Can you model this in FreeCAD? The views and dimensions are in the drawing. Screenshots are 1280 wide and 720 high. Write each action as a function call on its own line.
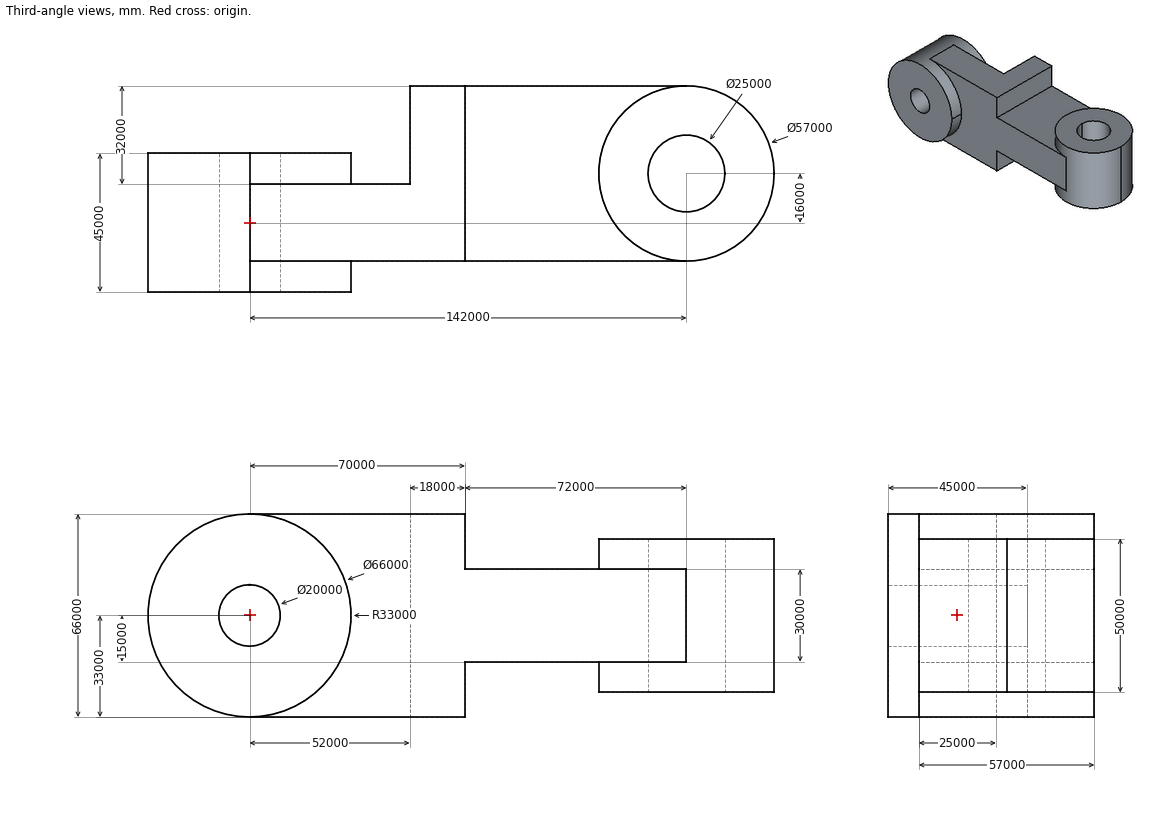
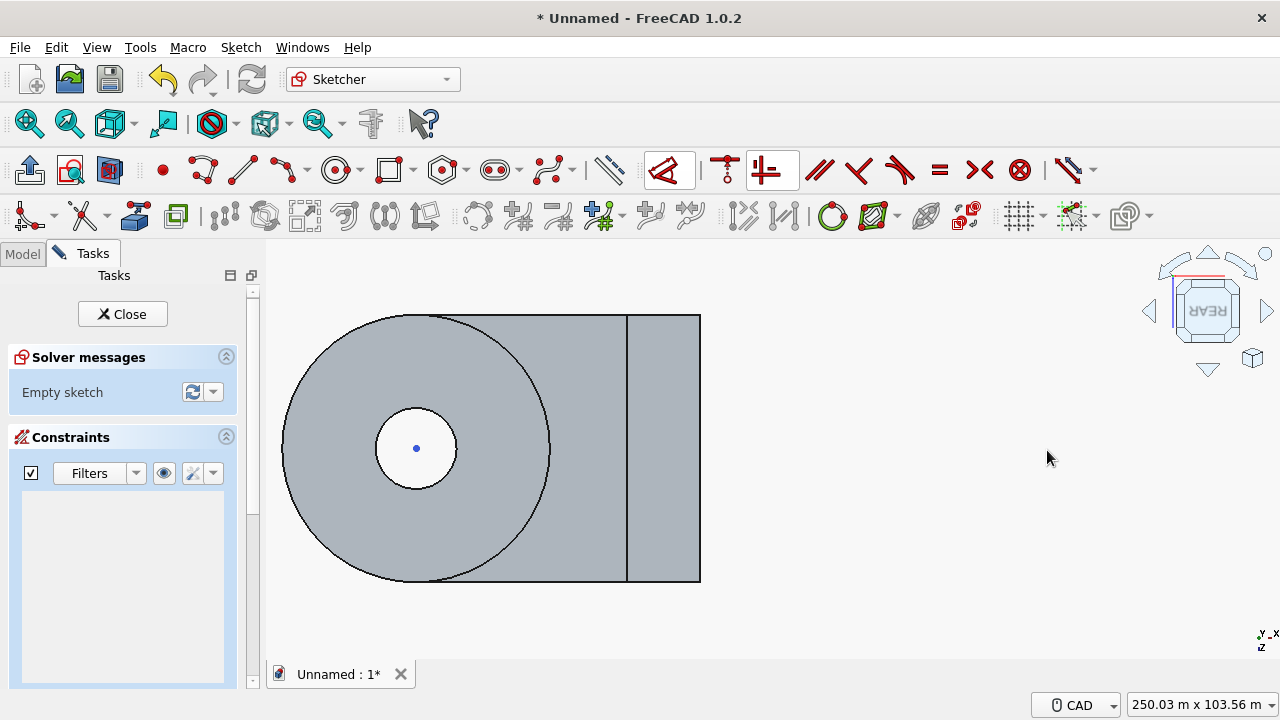
key(g)
key(r)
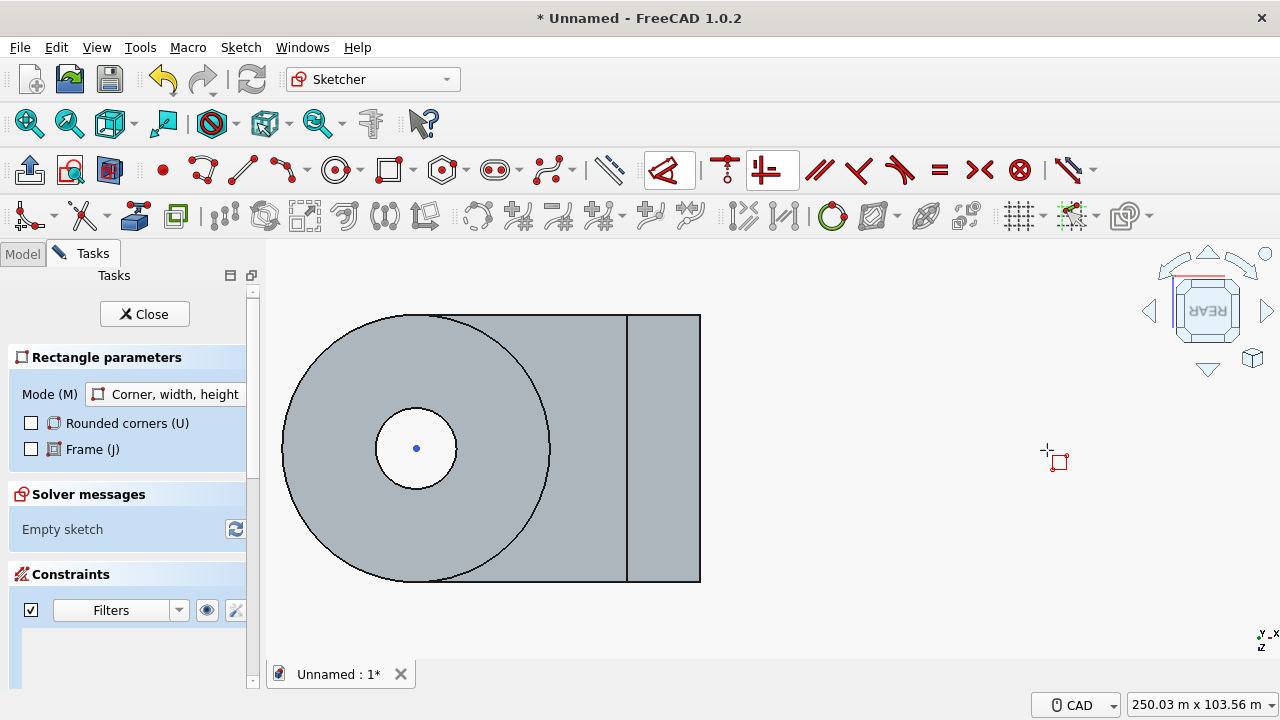
click(700, 388)
click(992, 509)
key(Escape)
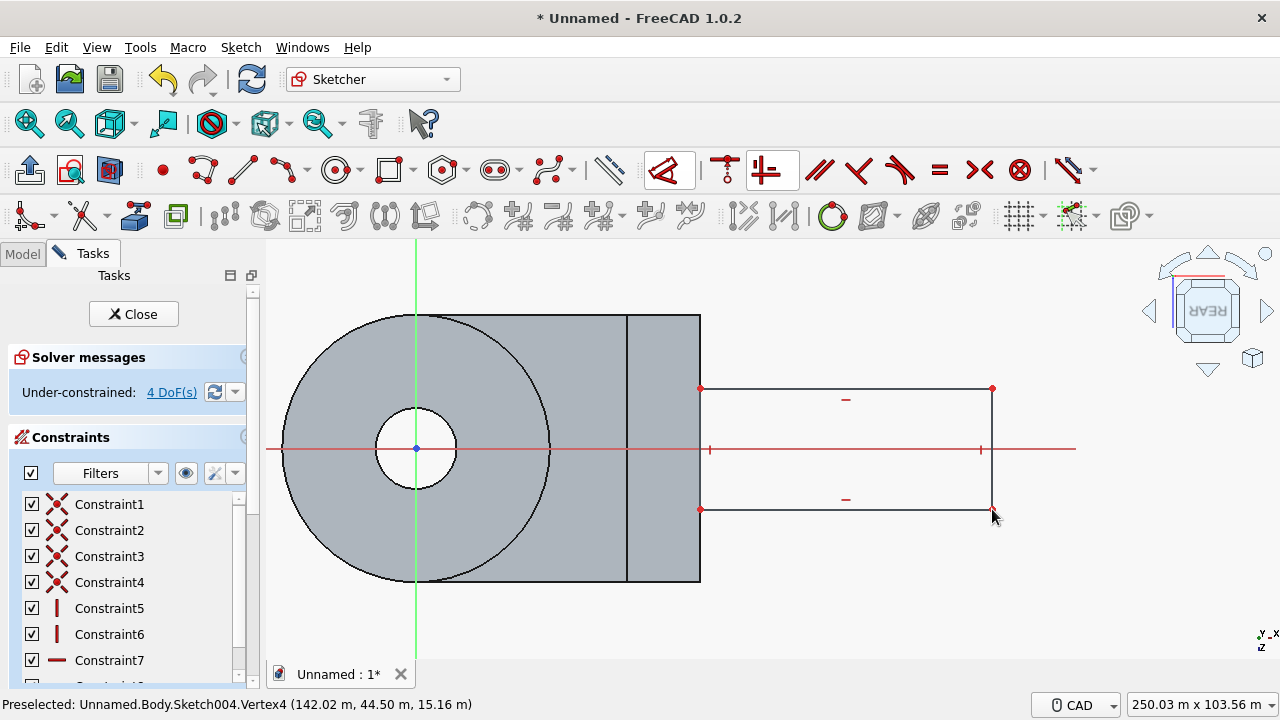
click(664, 170)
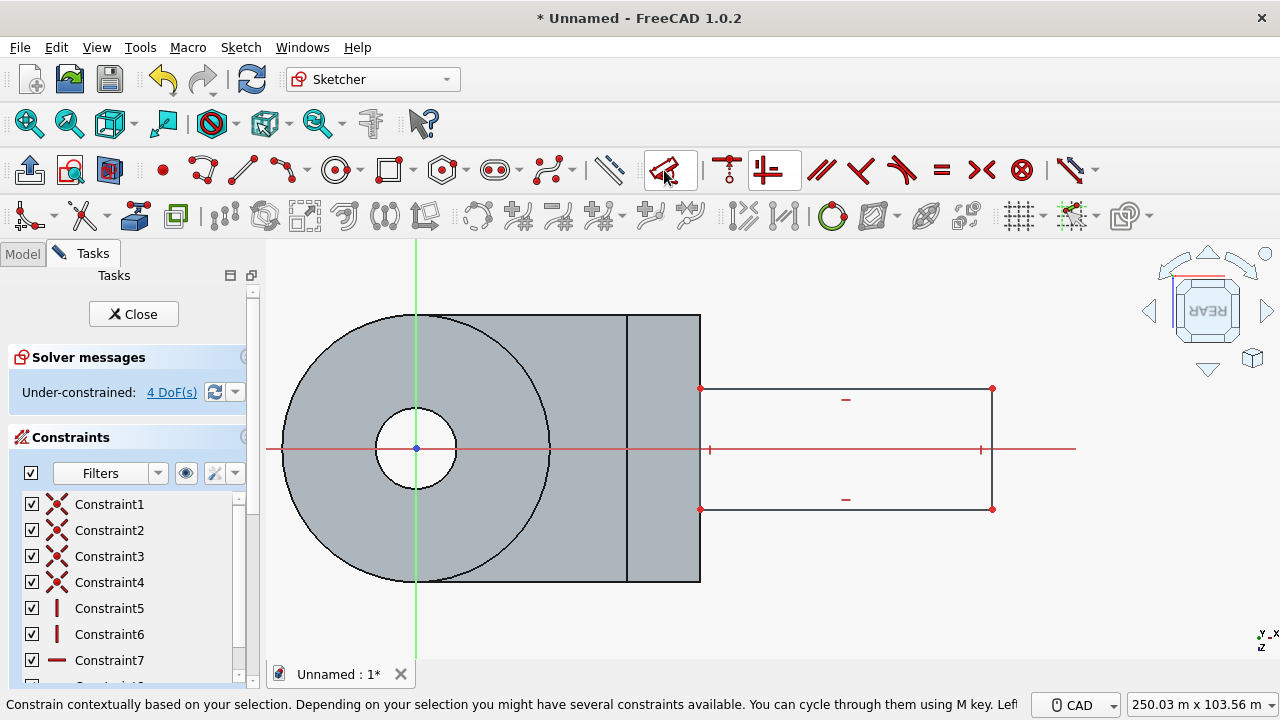
click(700, 425)
click(666, 422)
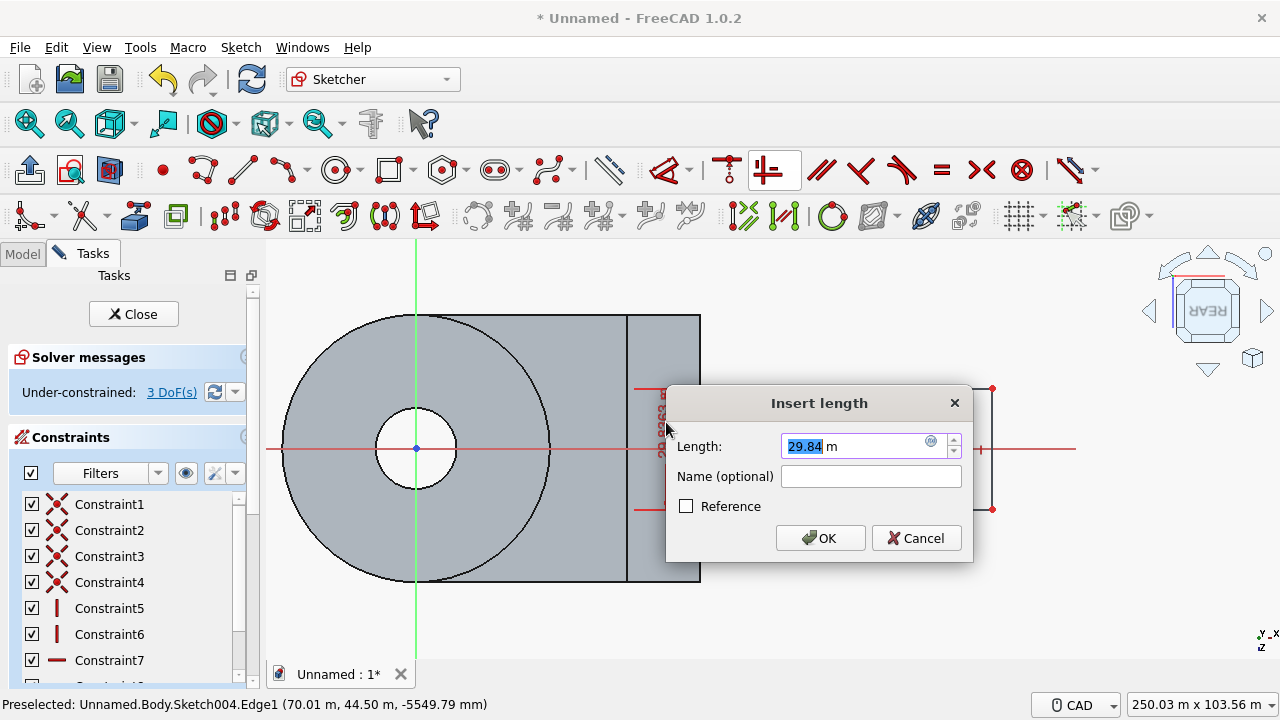
key(ctrl+a)
text(30000 mm)
key(Return)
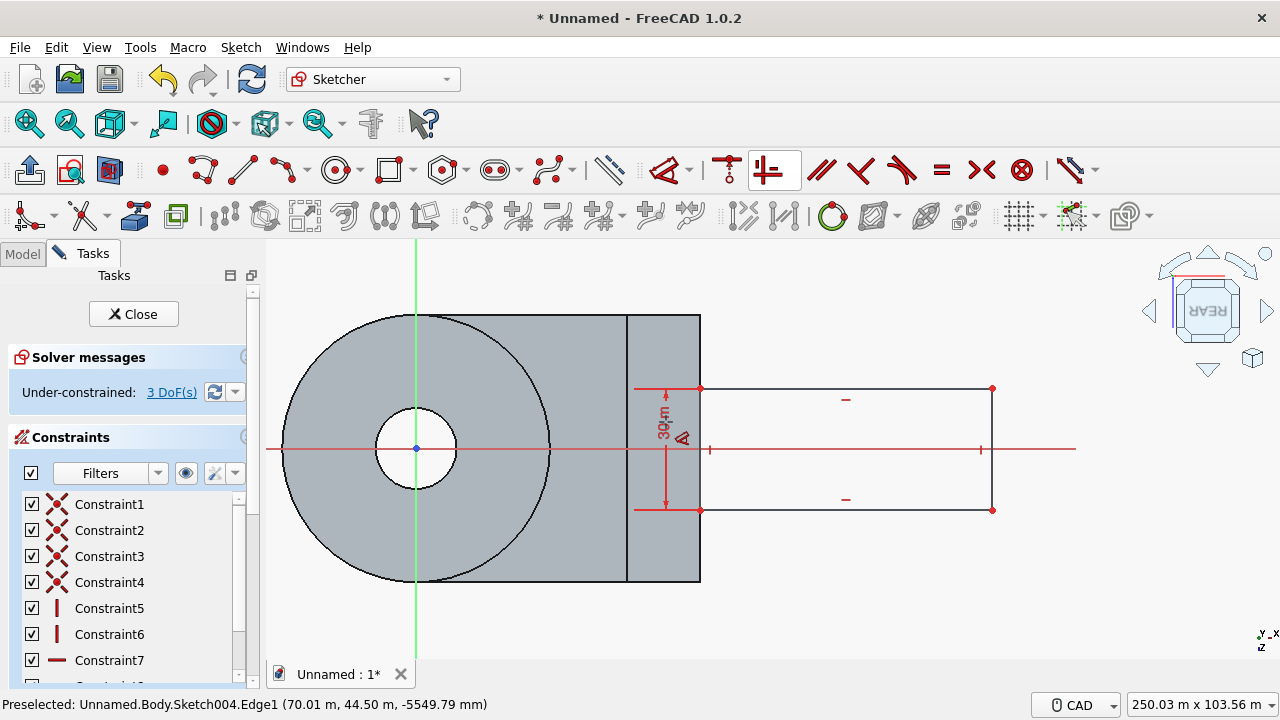
click(788, 510)
click(846, 544)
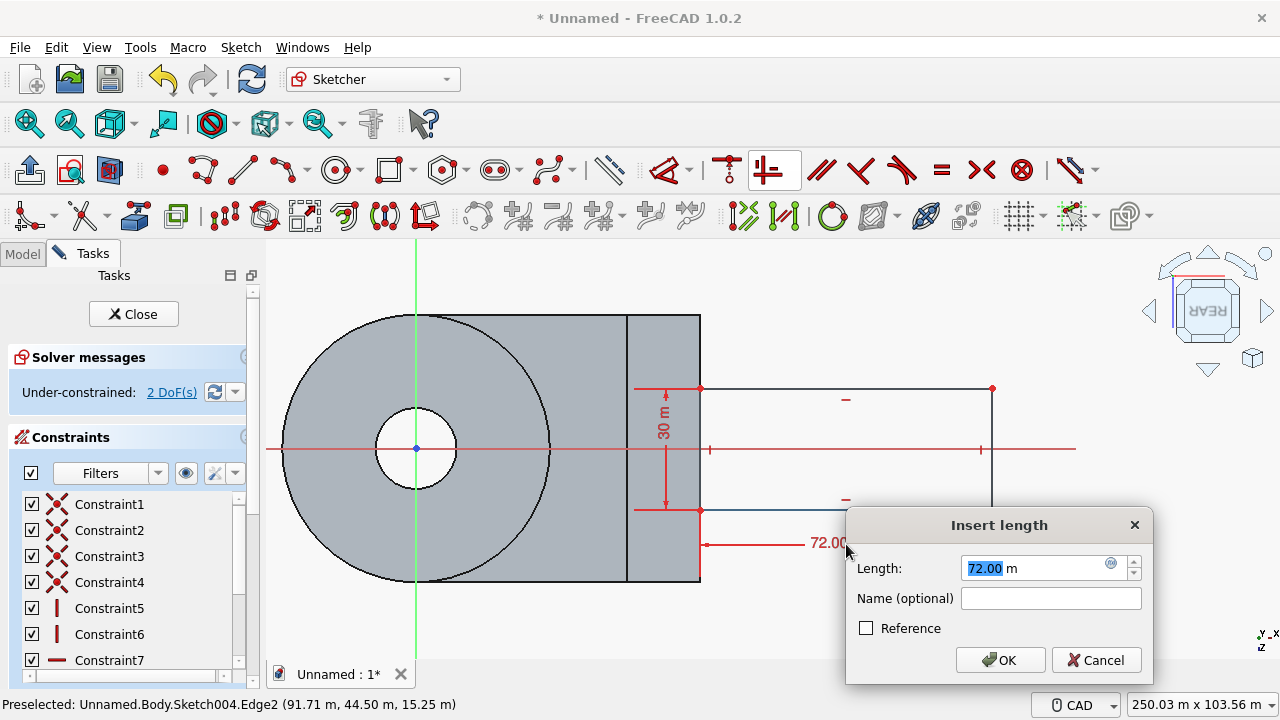
key(ctrl+a)
text(72000 mm)
key(Return)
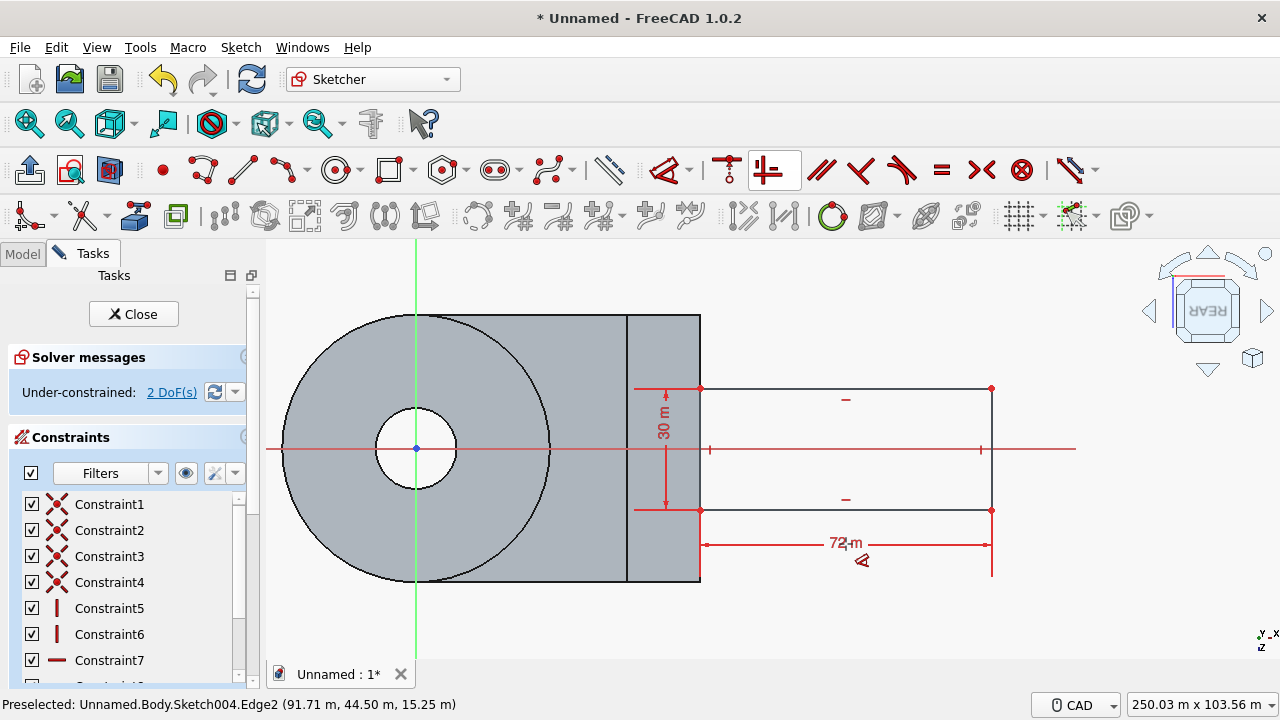
click(700, 389)
click(558, 355)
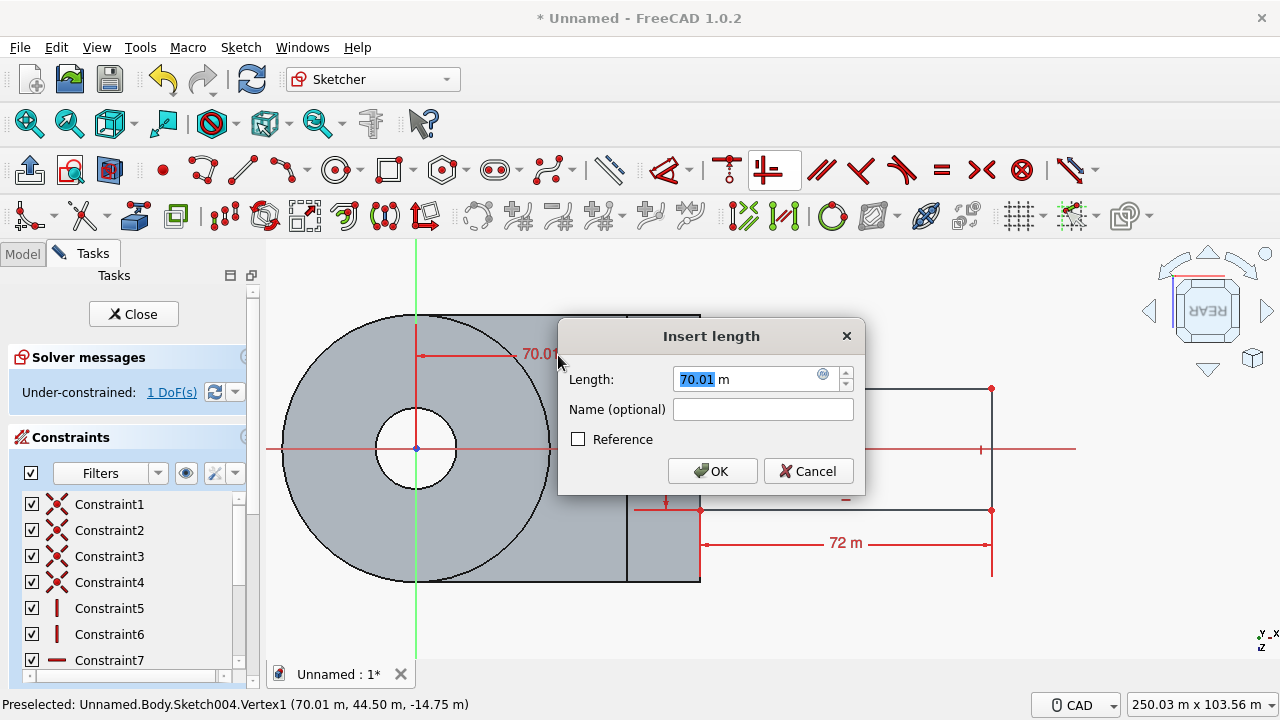
key(ctrl+a)
text(70000 mm)
key(Return)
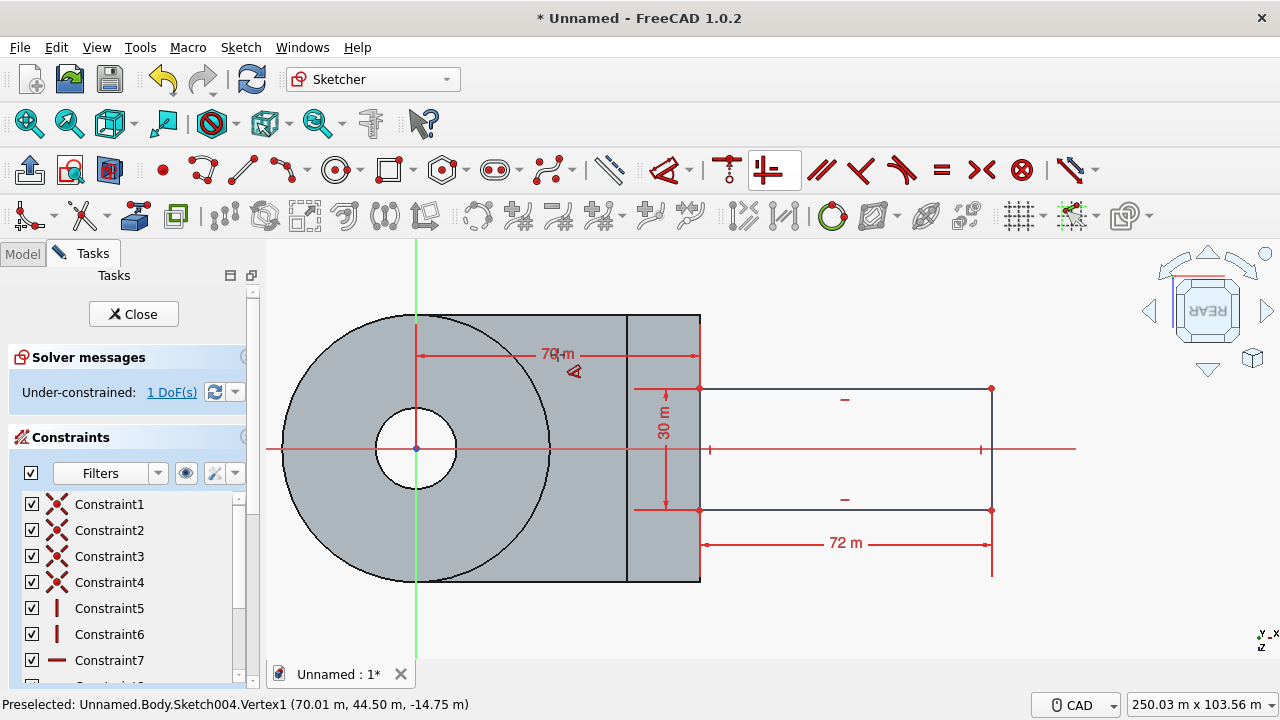
click(700, 389)
click(382, 419)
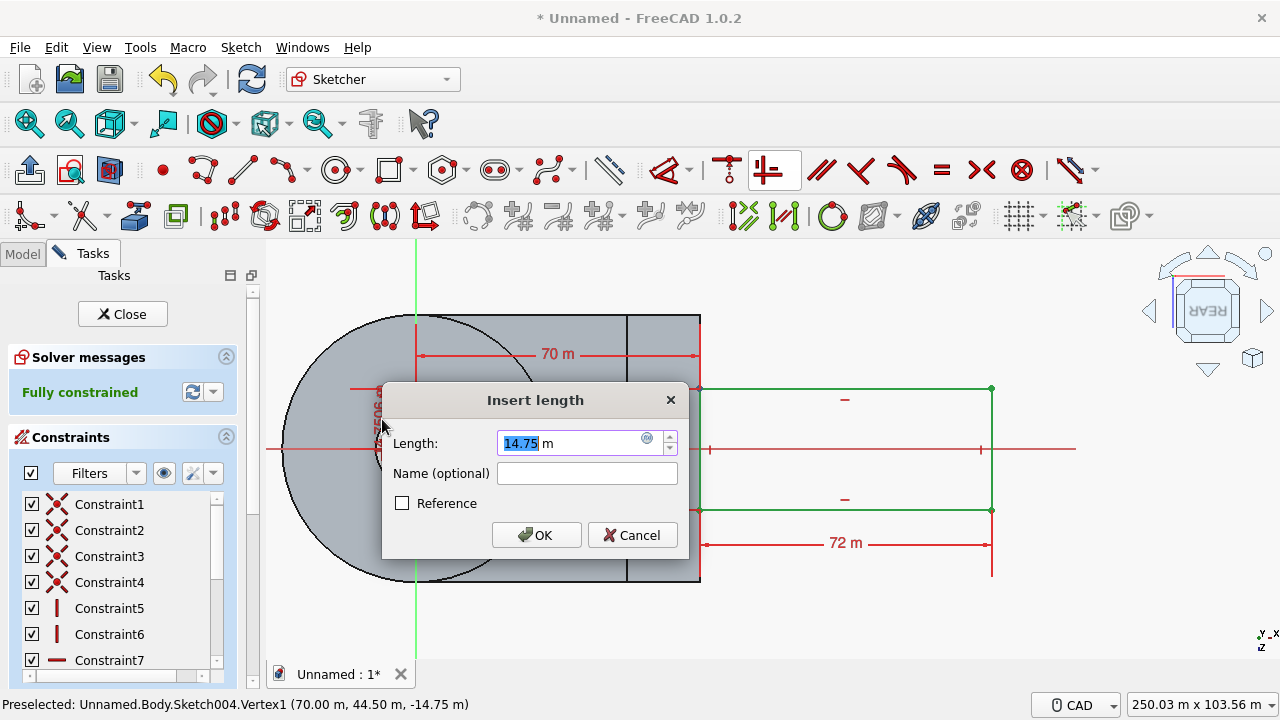
key(ctrl+a)
text(15000 mm)
key(Return)
key(Escape)